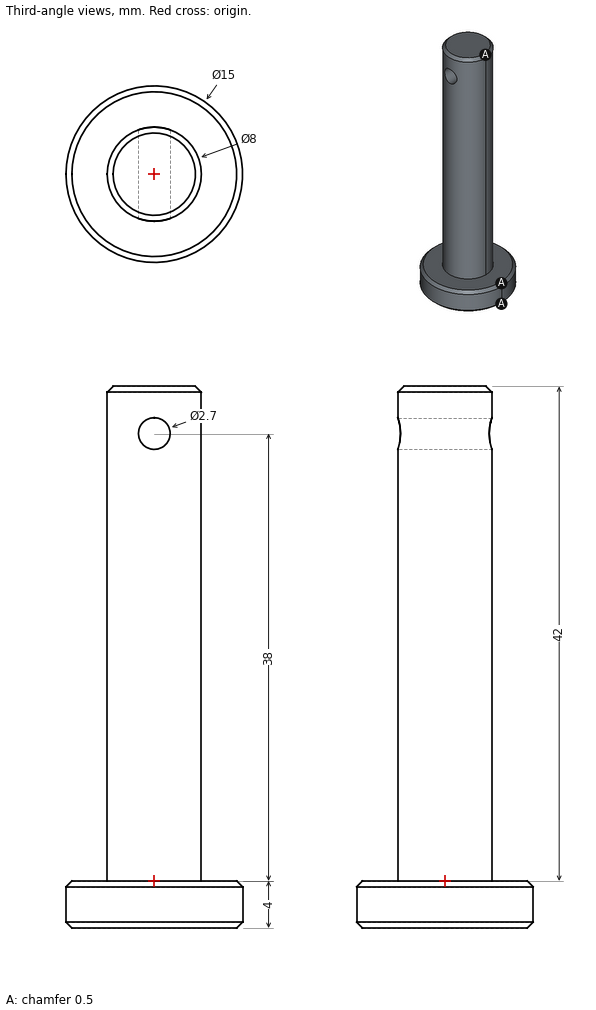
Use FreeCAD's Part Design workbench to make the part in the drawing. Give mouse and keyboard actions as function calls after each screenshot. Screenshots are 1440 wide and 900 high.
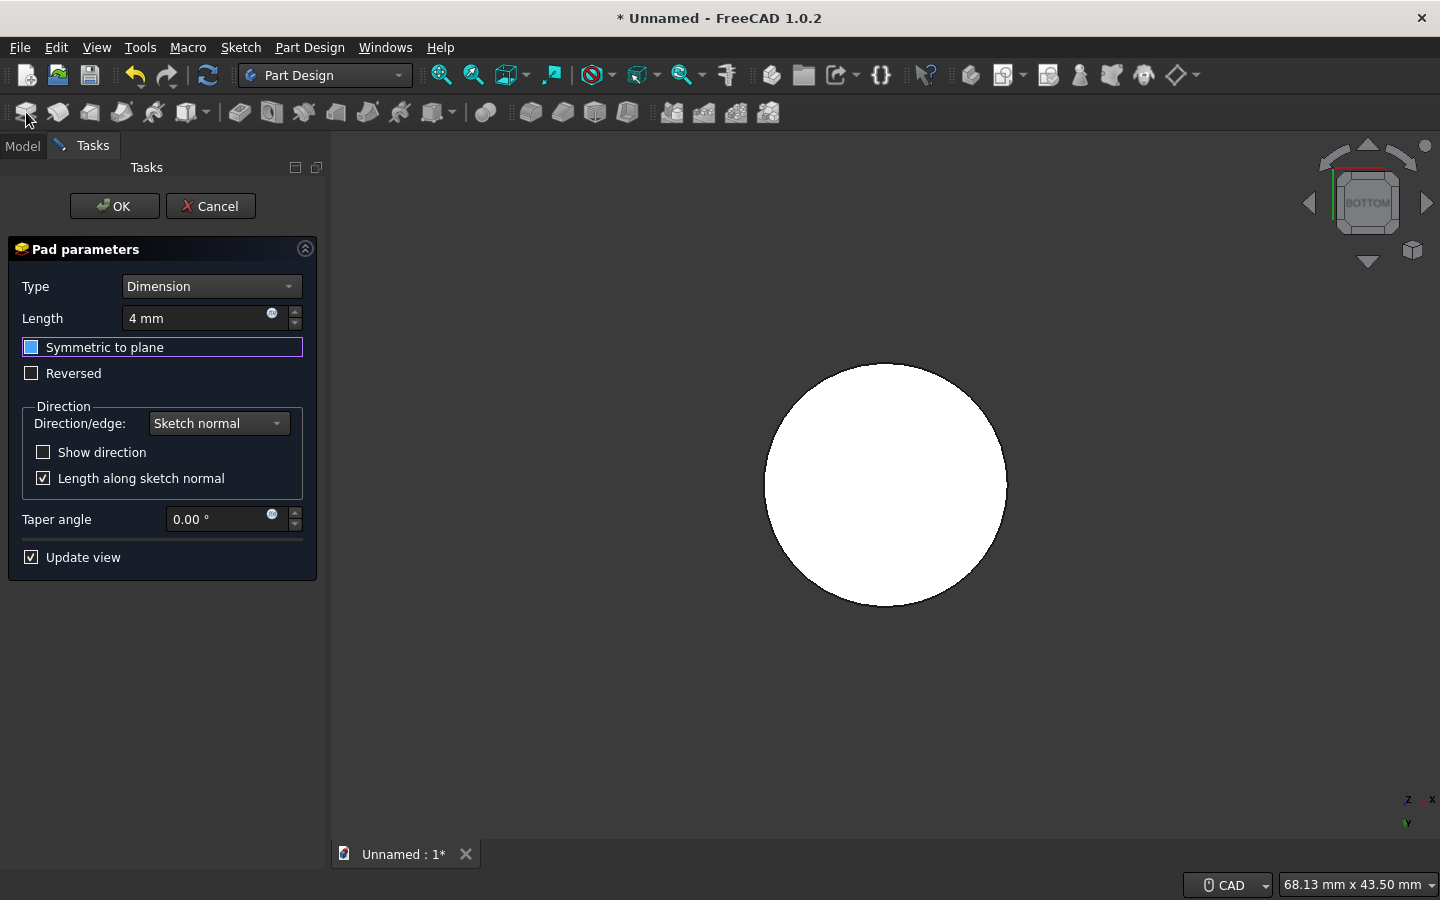
click(115, 206)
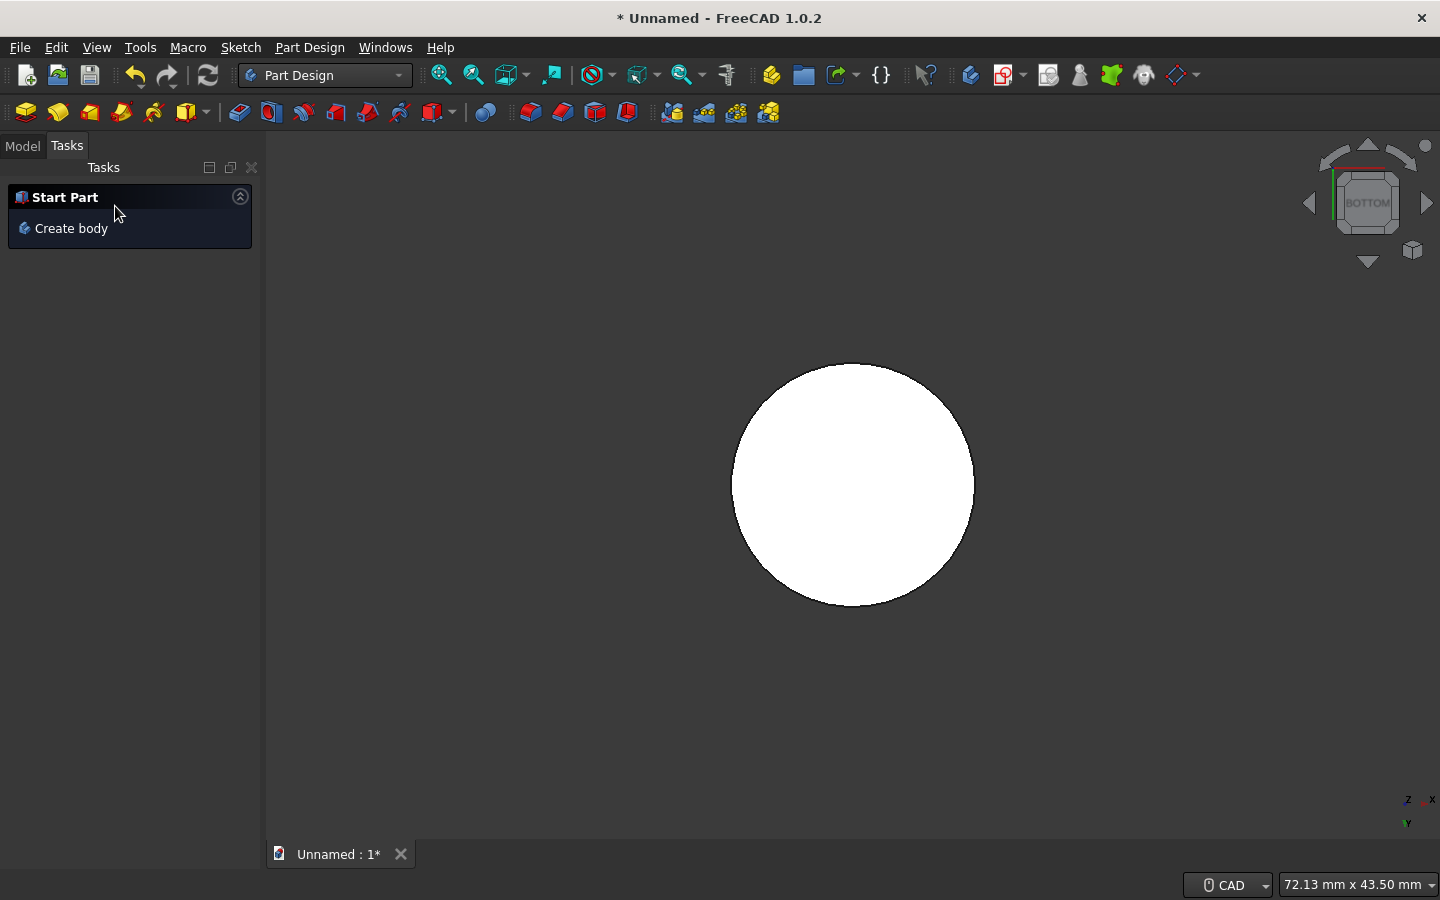
click(442, 76)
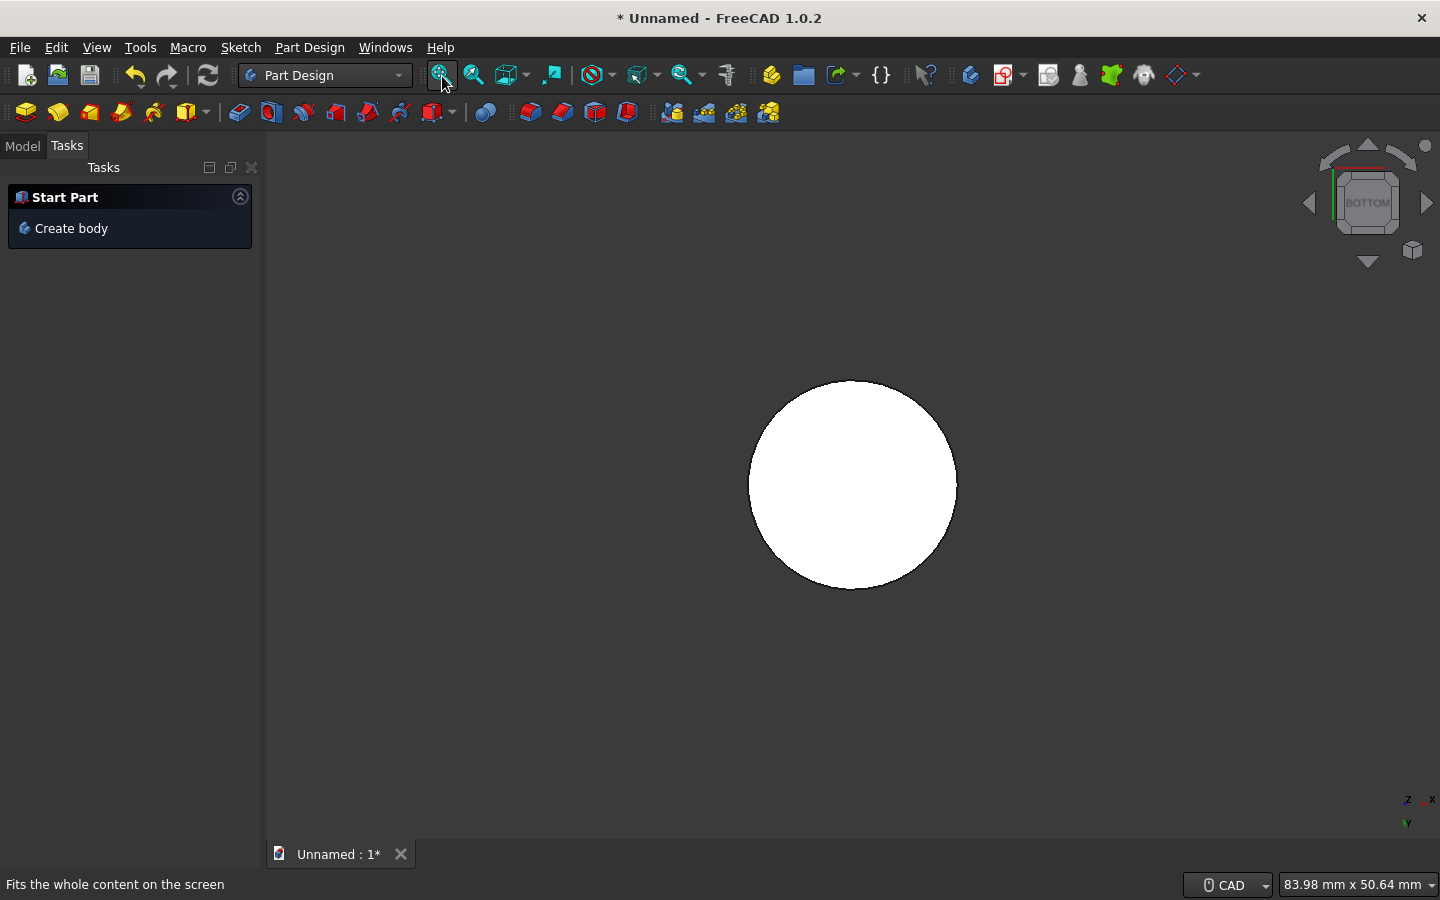
click(1004, 76)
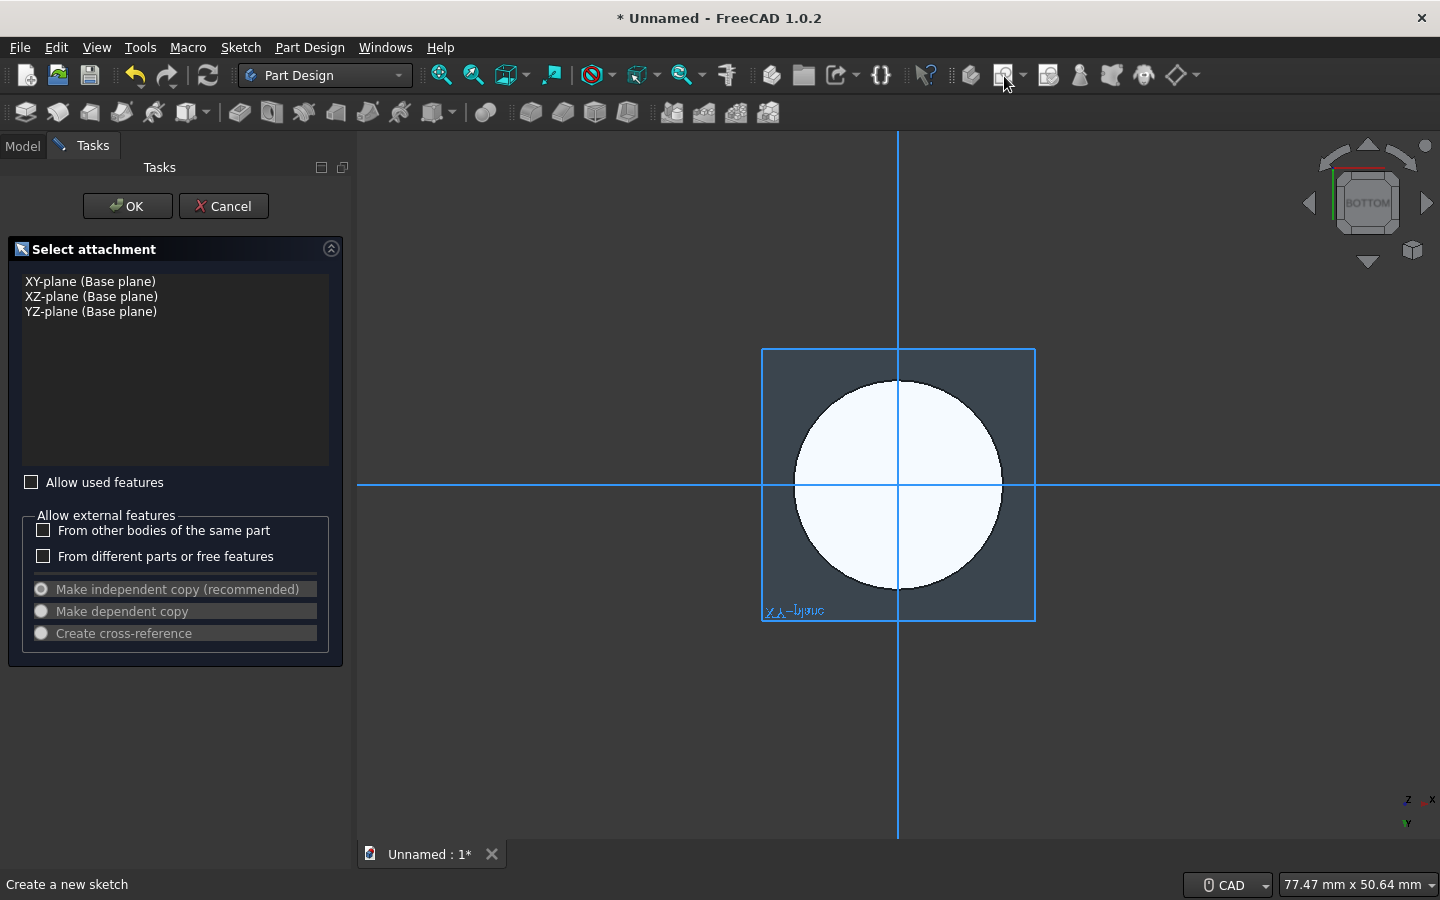
click(82, 296)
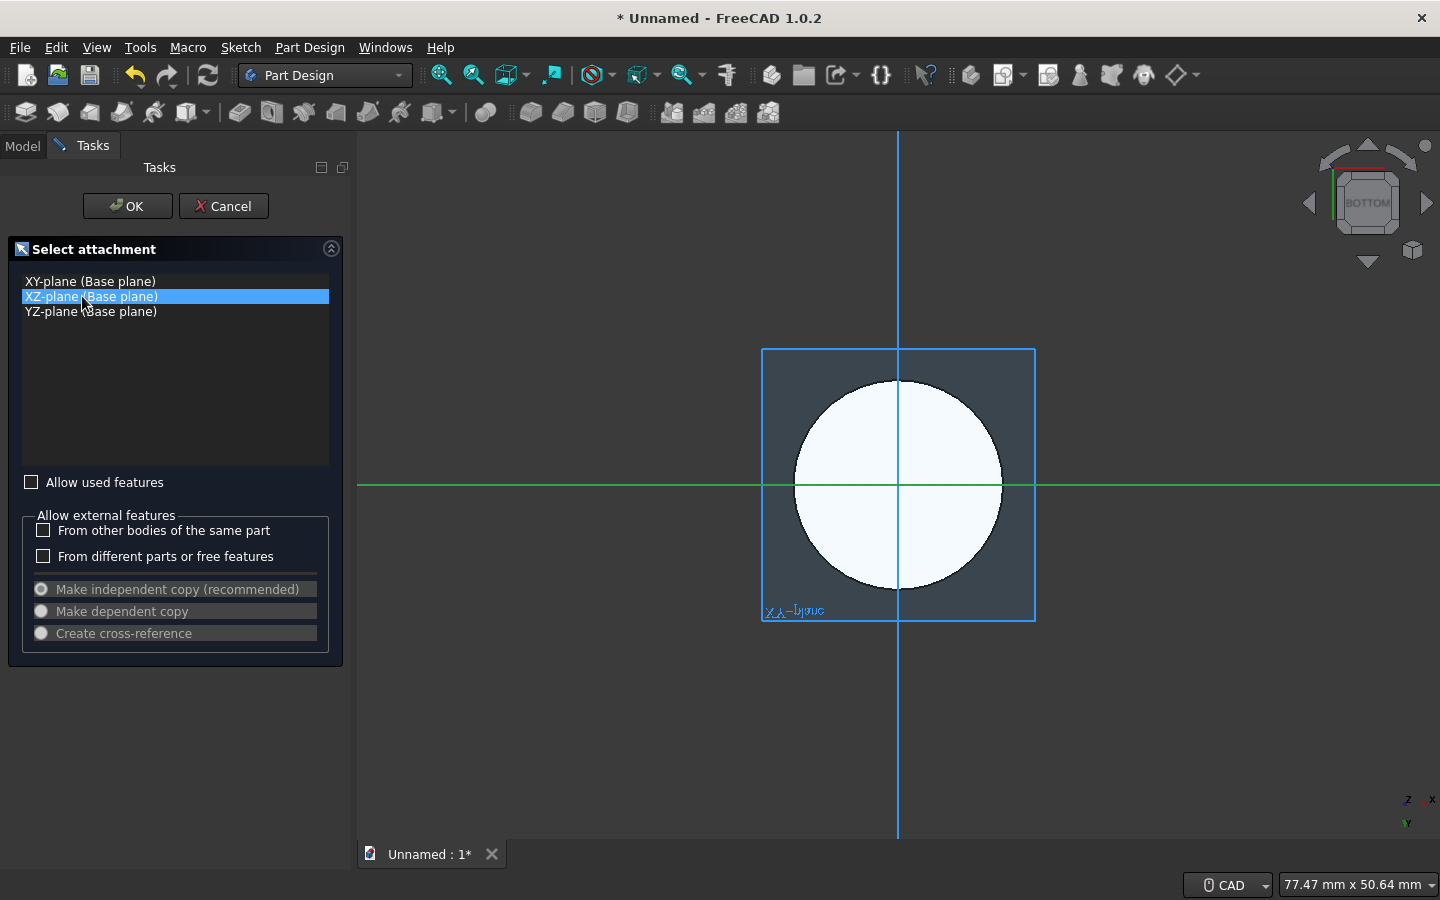
click(128, 206)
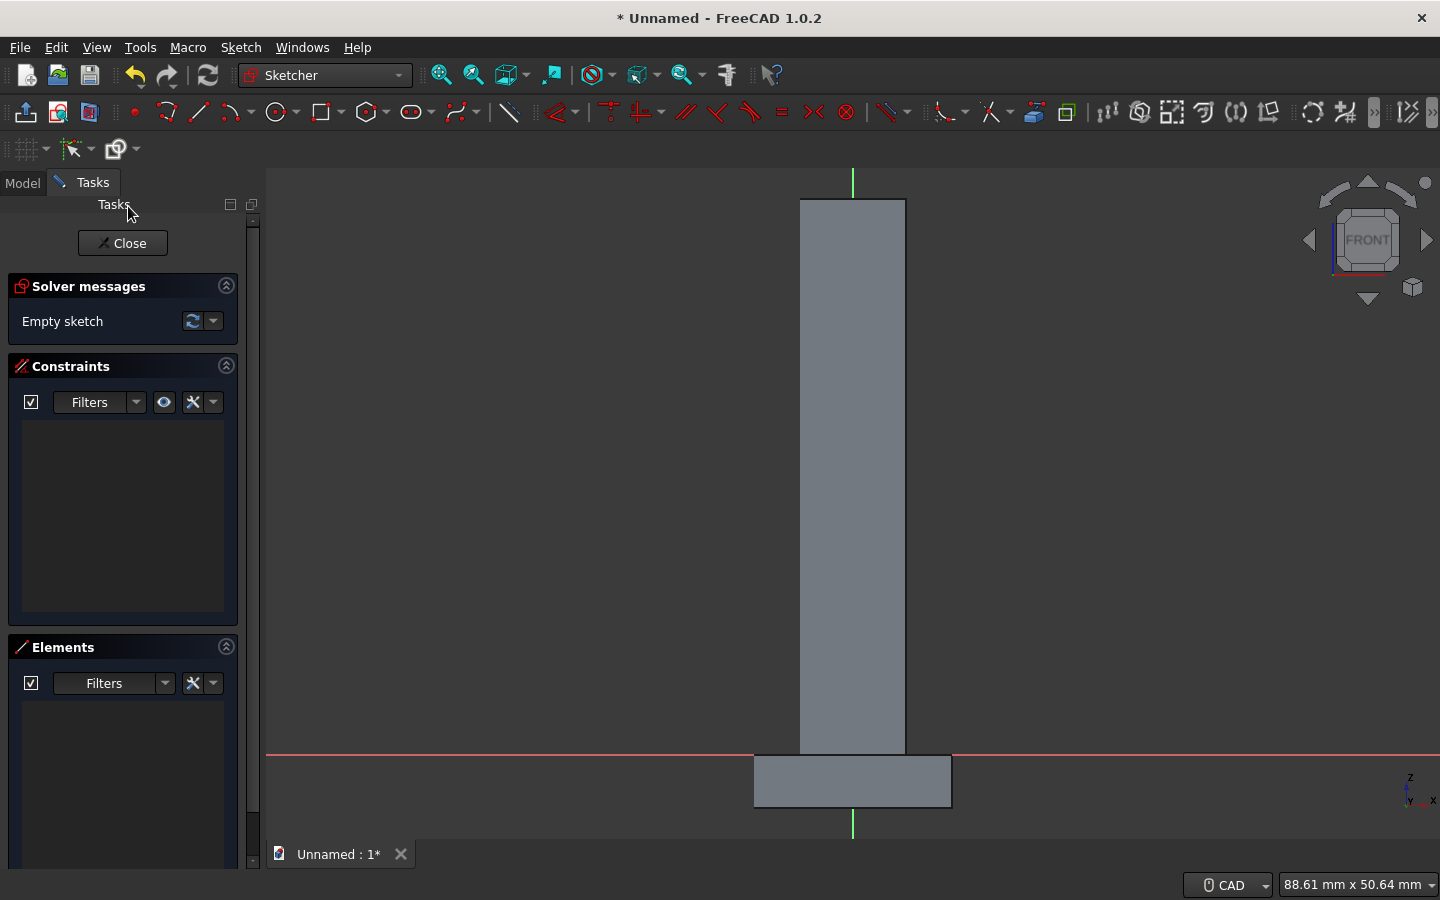
click(90, 112)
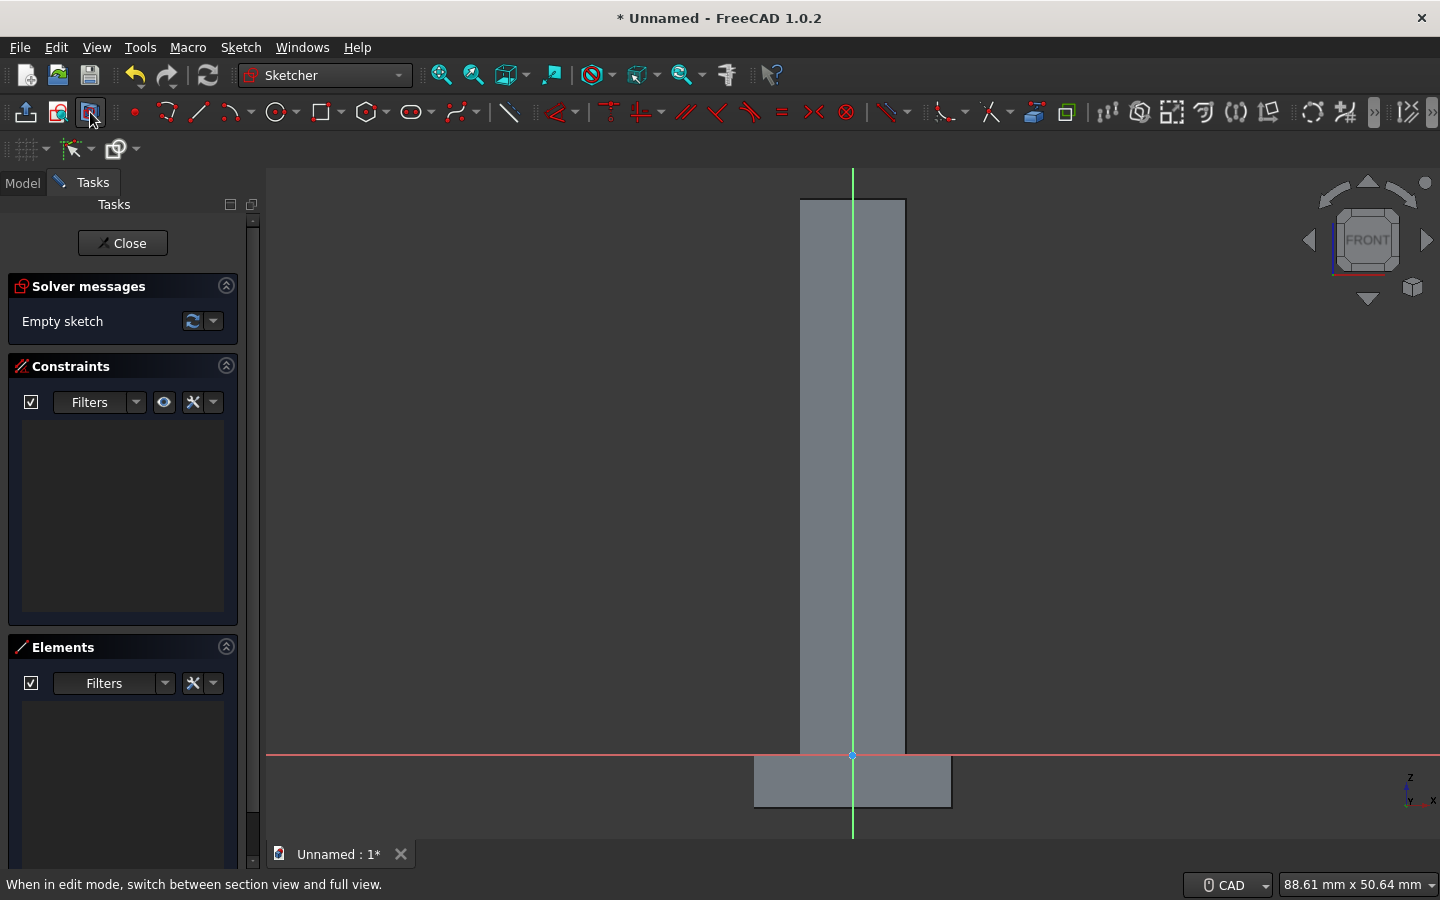
scroll(860, 227, up, 12)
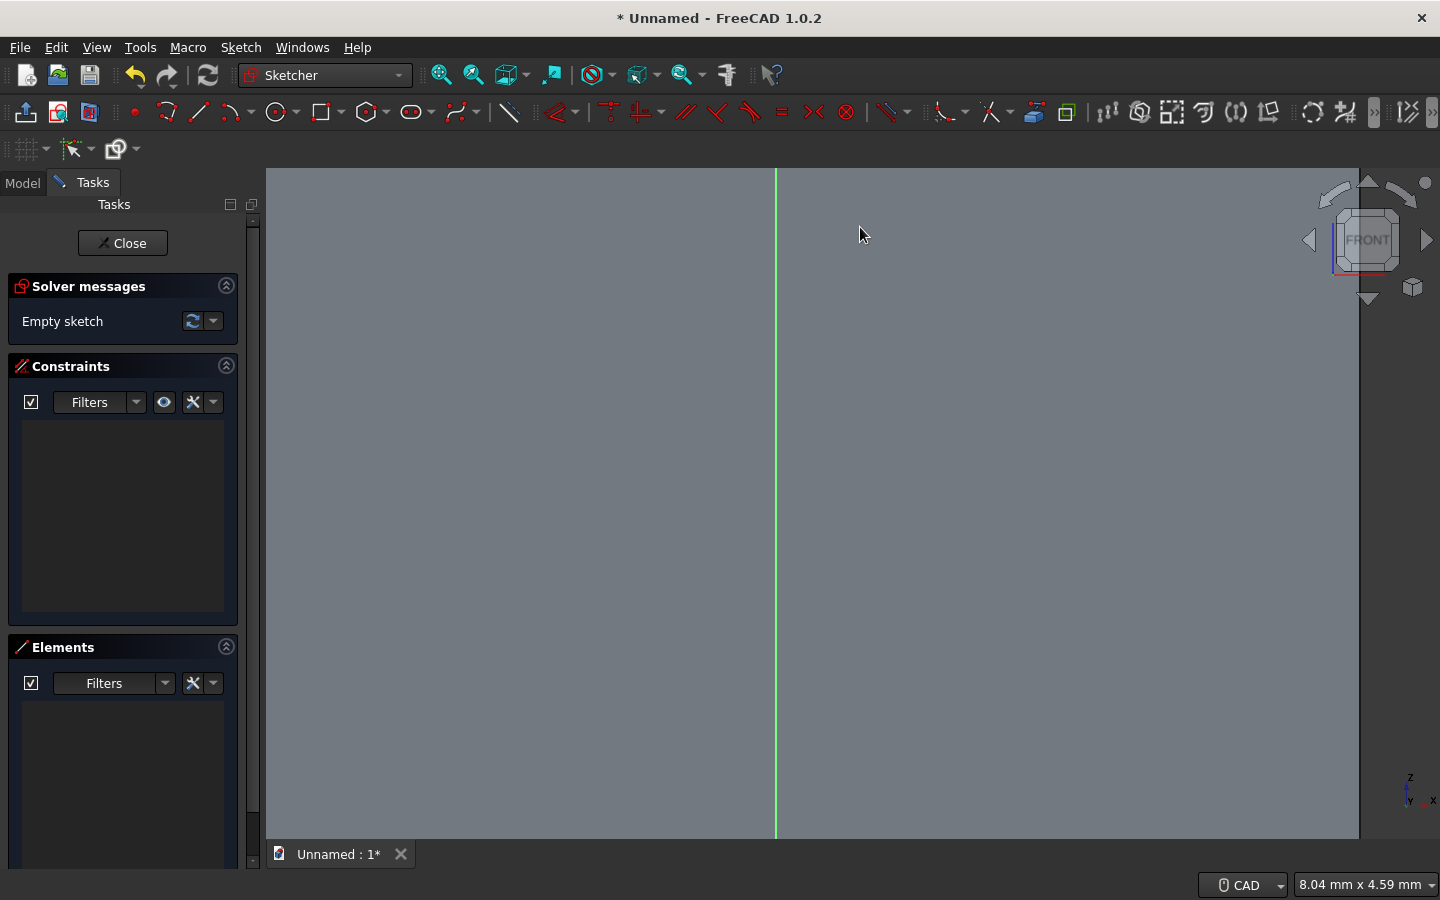
click(276, 112)